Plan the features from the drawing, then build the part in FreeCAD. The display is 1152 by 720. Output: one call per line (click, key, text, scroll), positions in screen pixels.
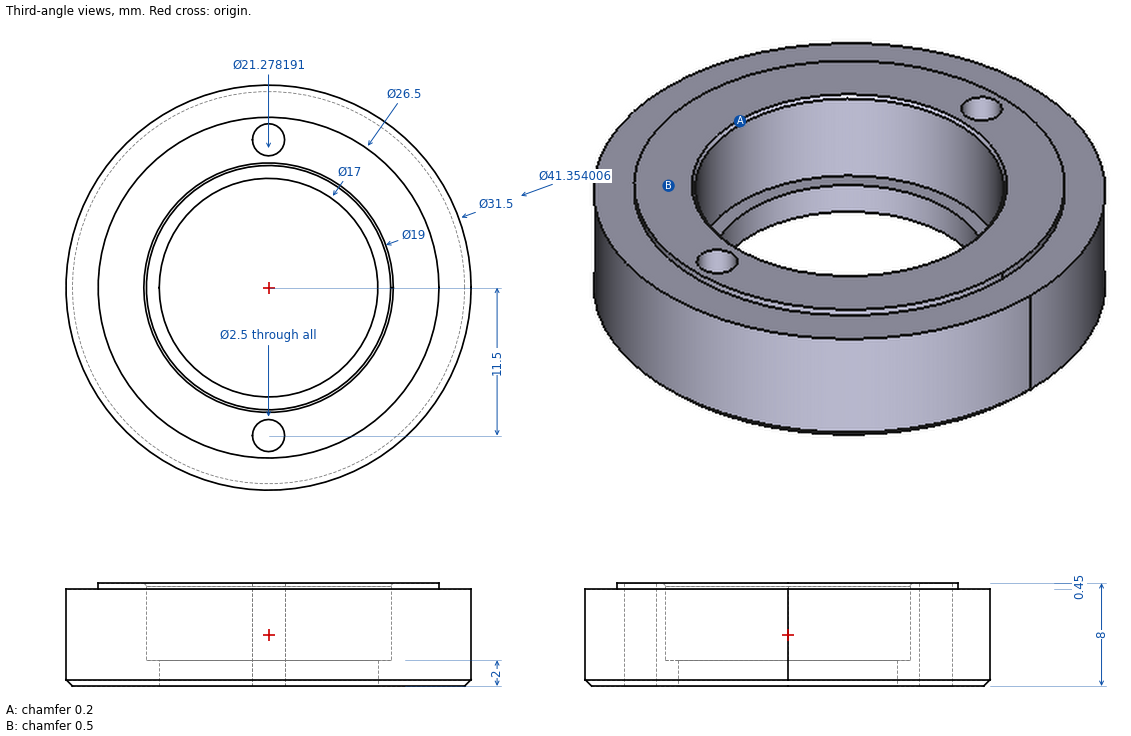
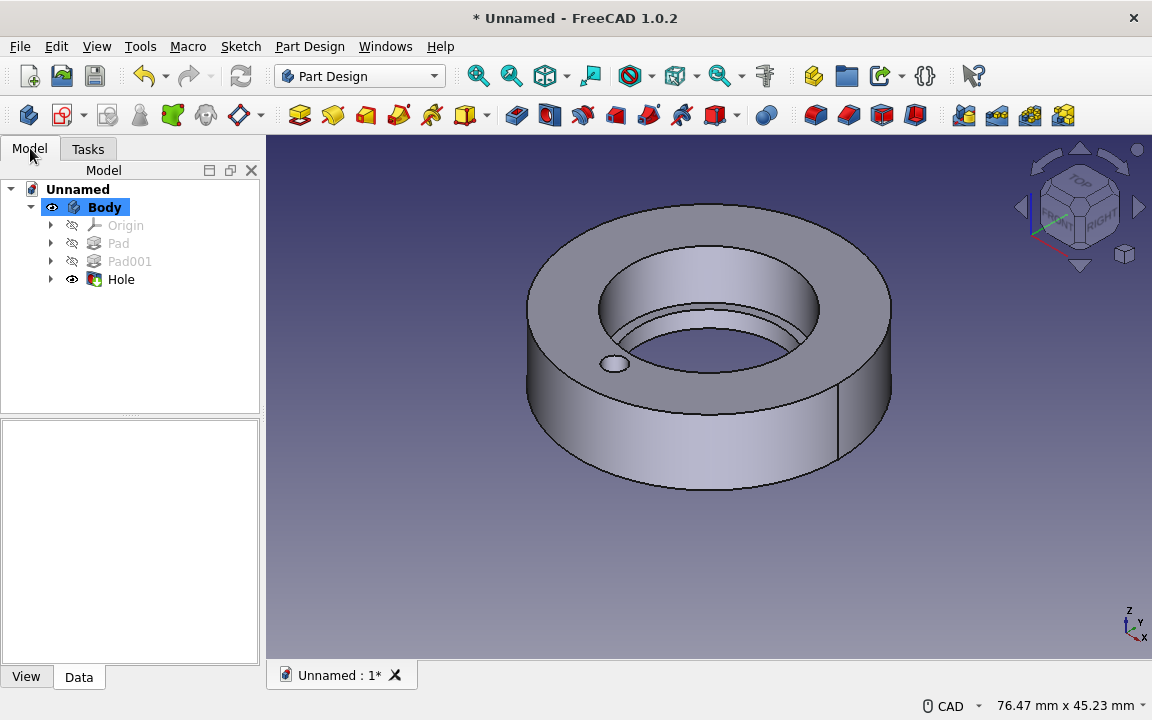
click(117, 279)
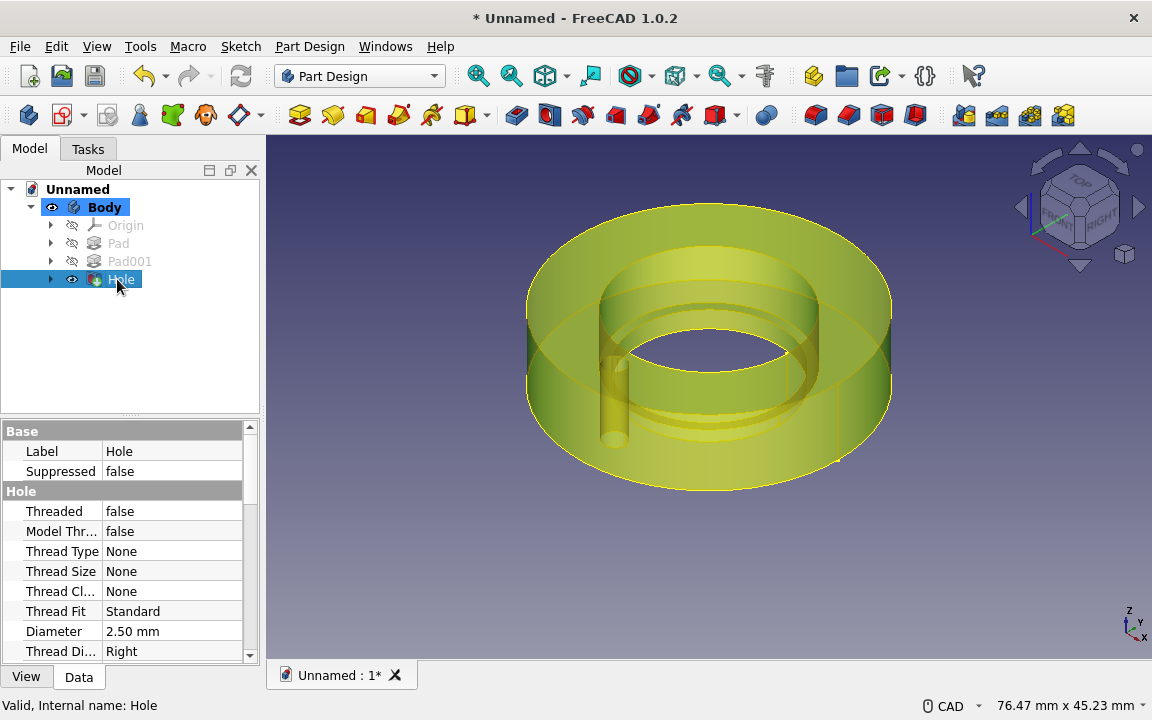
click(964, 116)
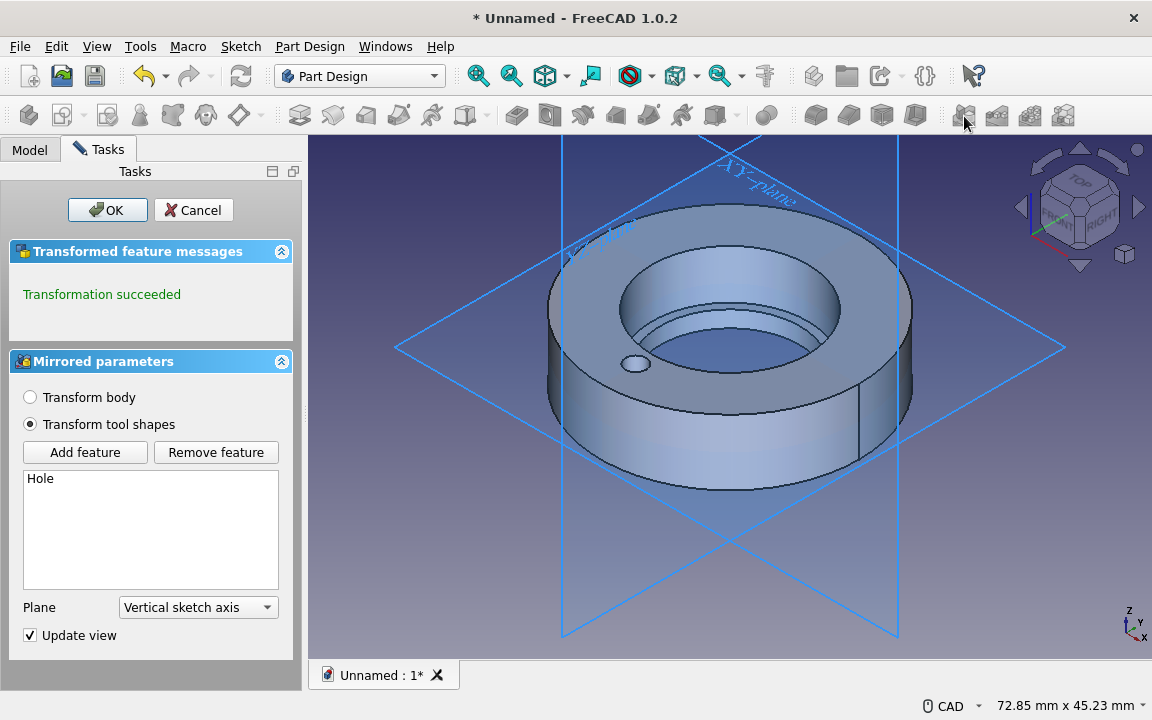
click(199, 608)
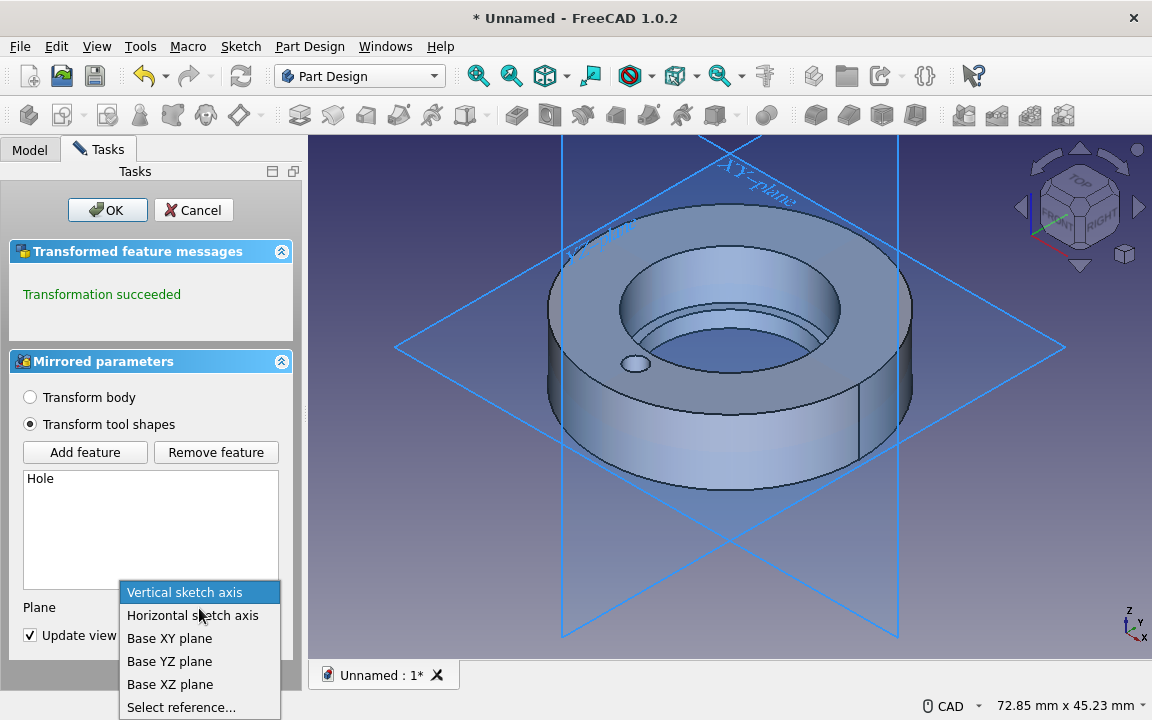
click(198, 684)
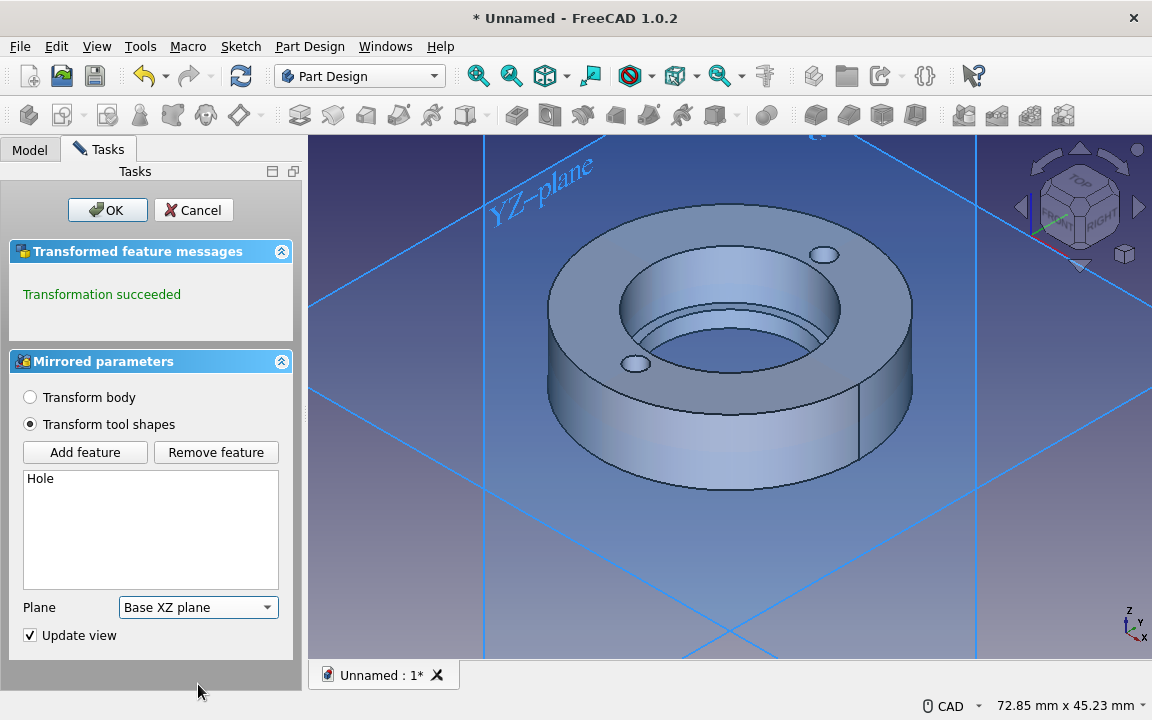
click(108, 210)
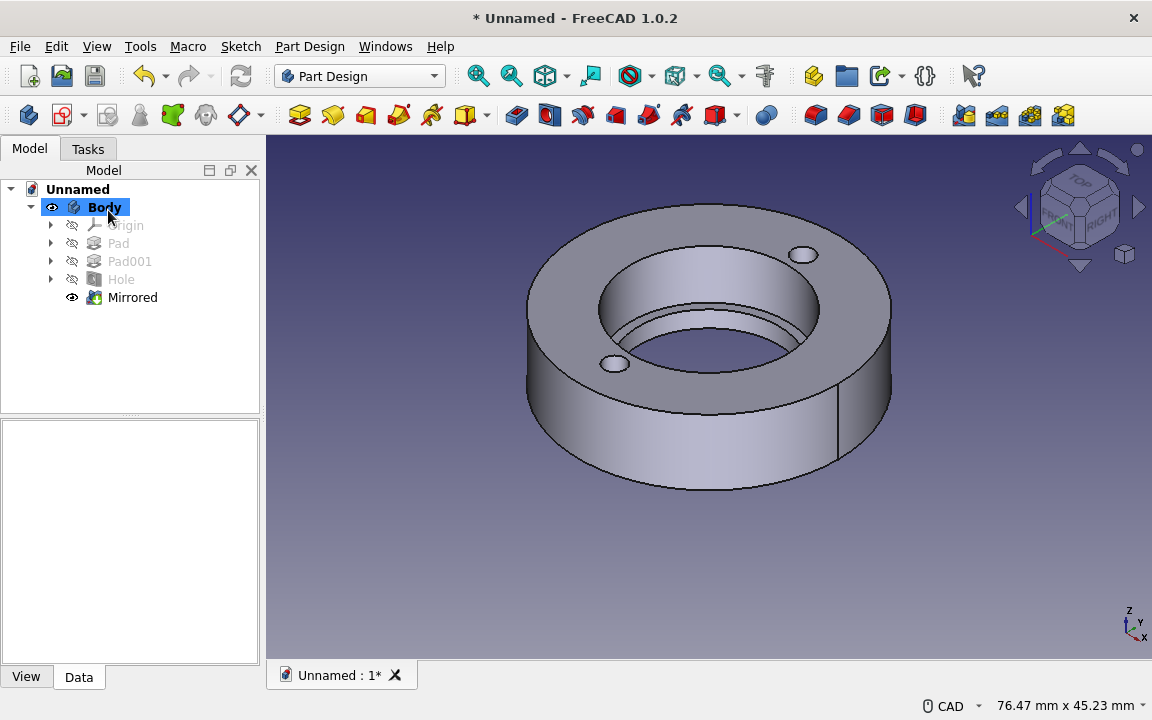
click(631, 263)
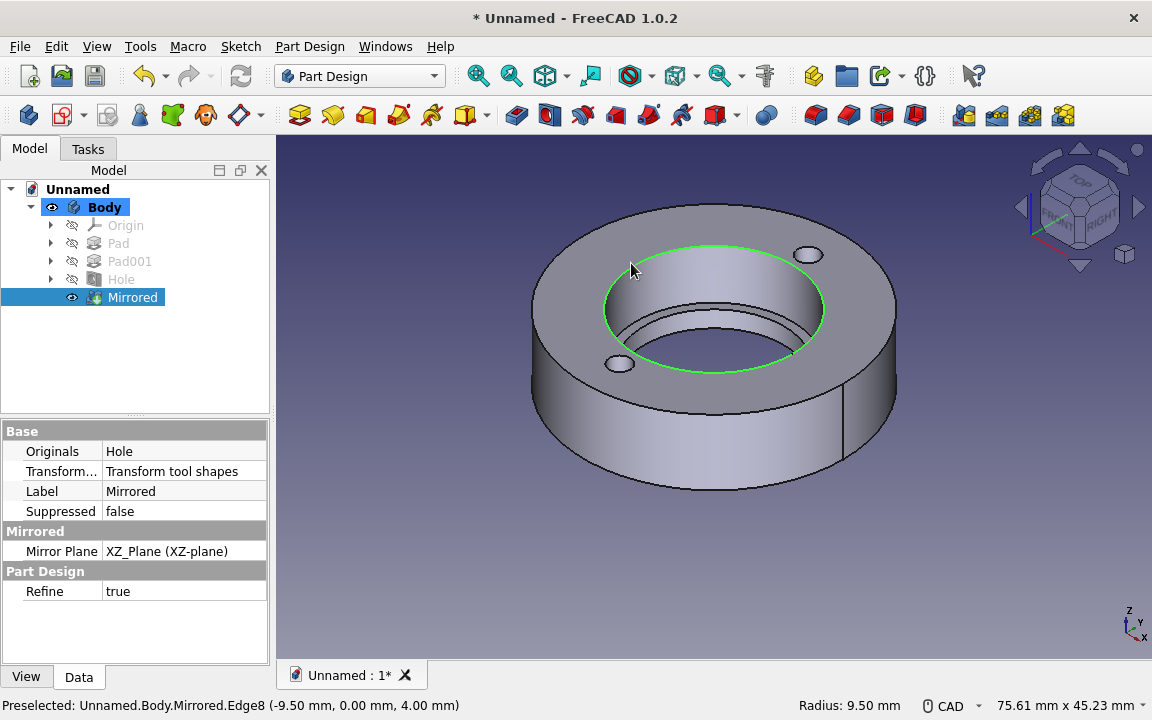
click(849, 116)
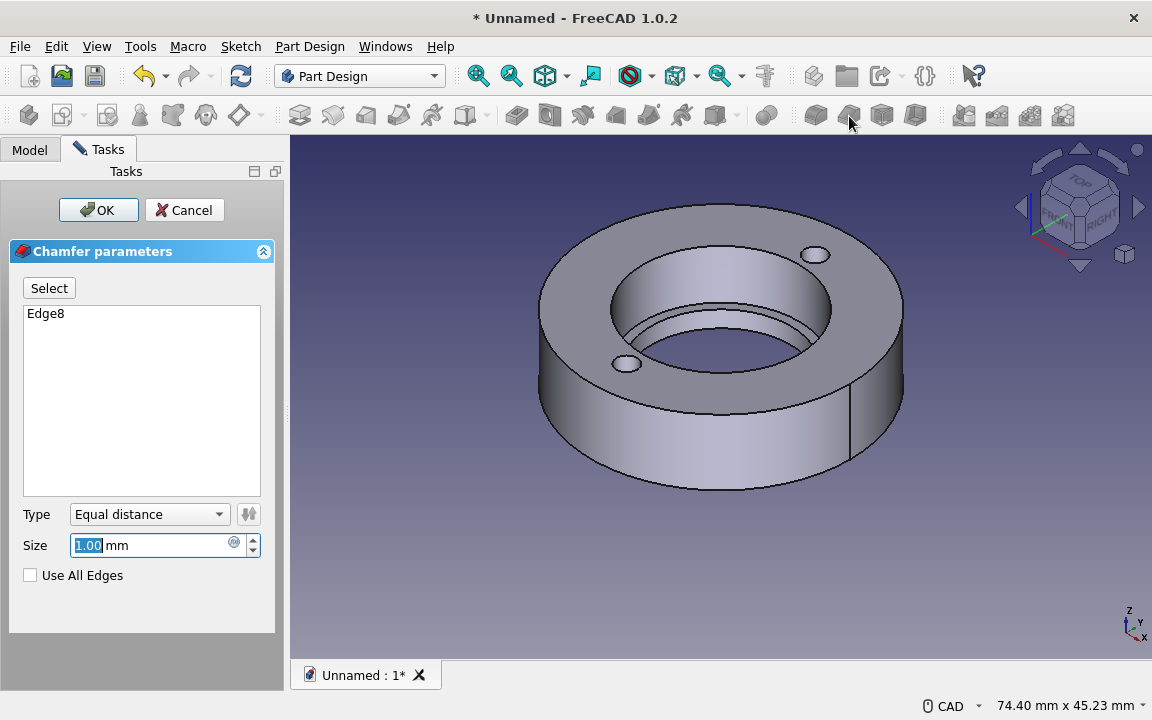
text(0.2)
key(Tab)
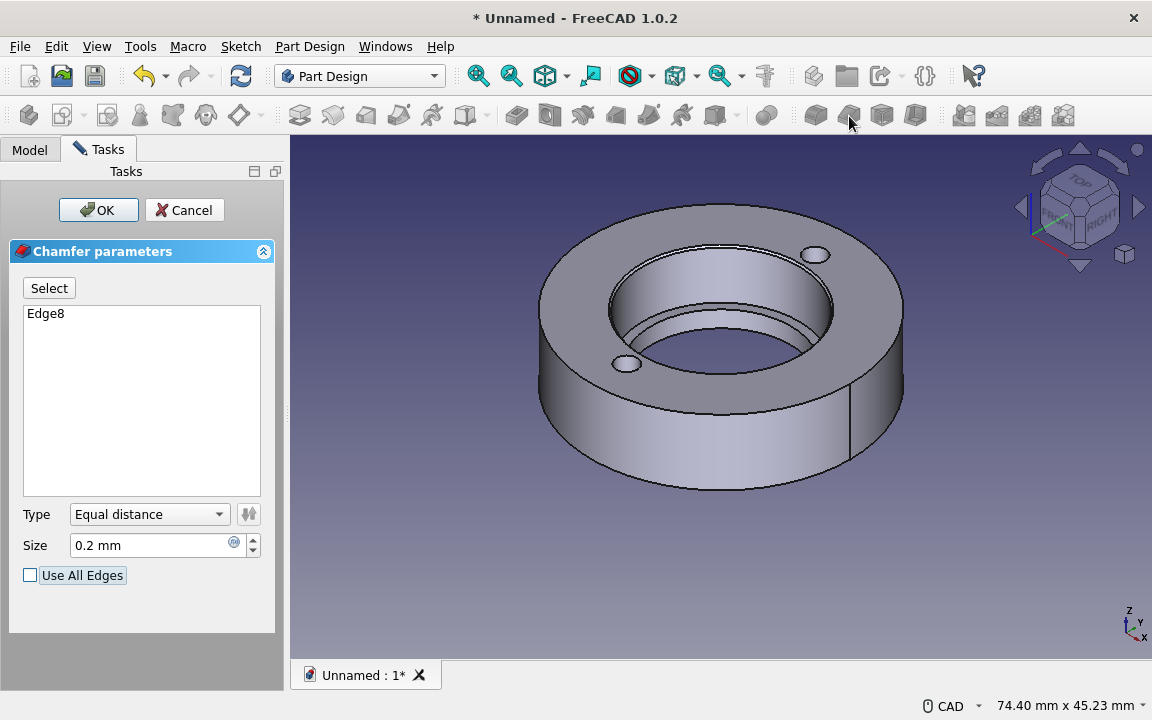
click(99, 210)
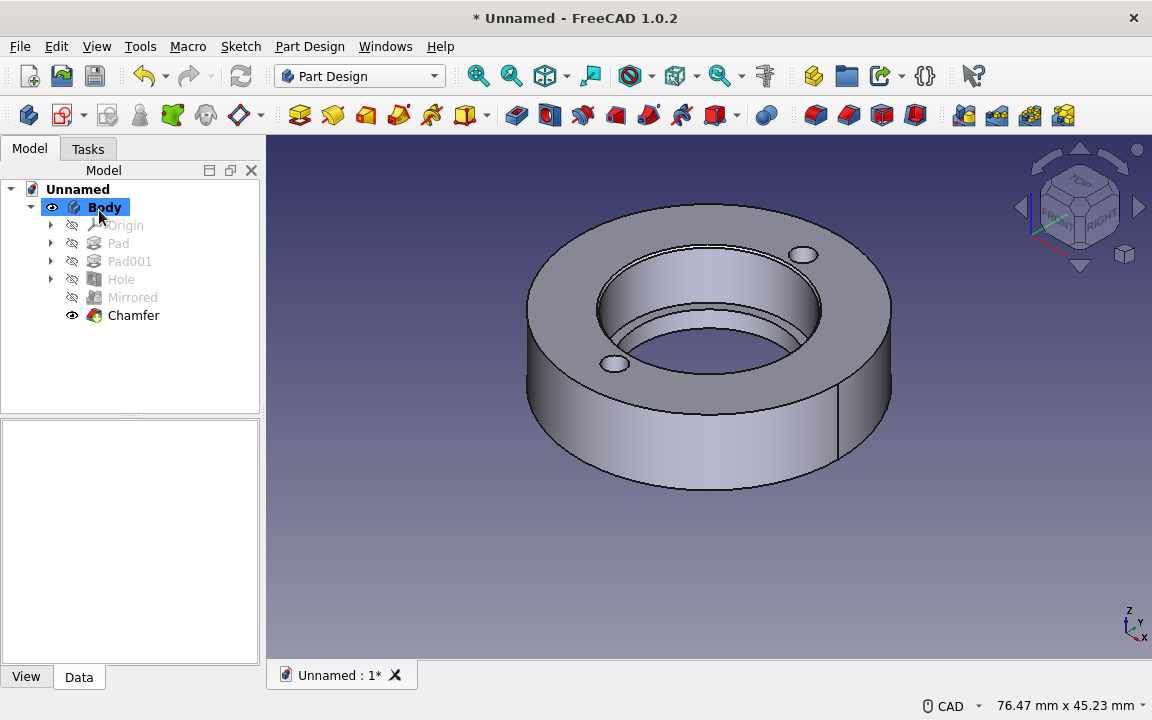
click(562, 308)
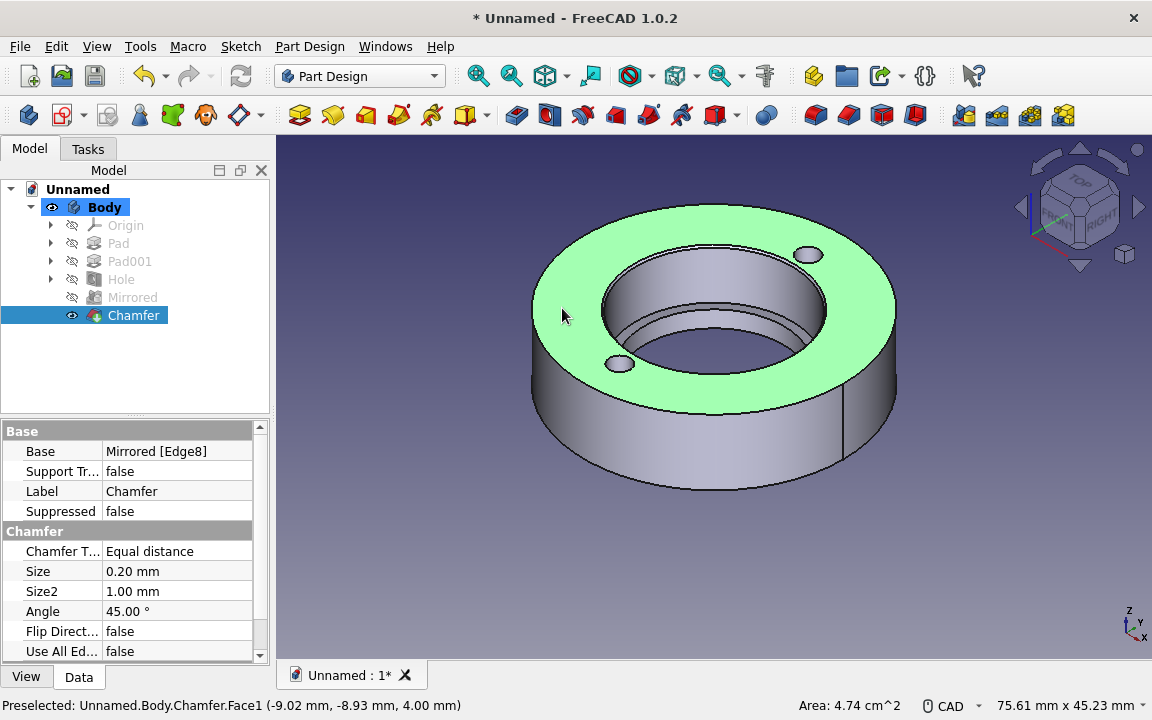
click(62, 116)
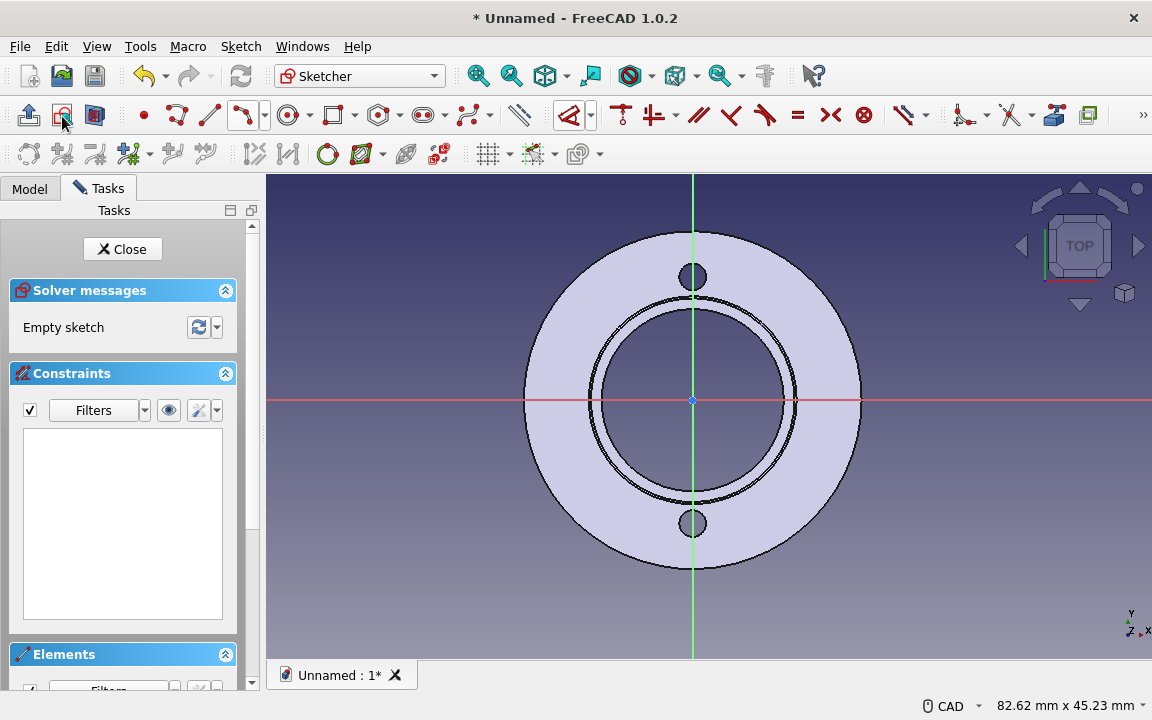
scroll(534, 450, down, 2)